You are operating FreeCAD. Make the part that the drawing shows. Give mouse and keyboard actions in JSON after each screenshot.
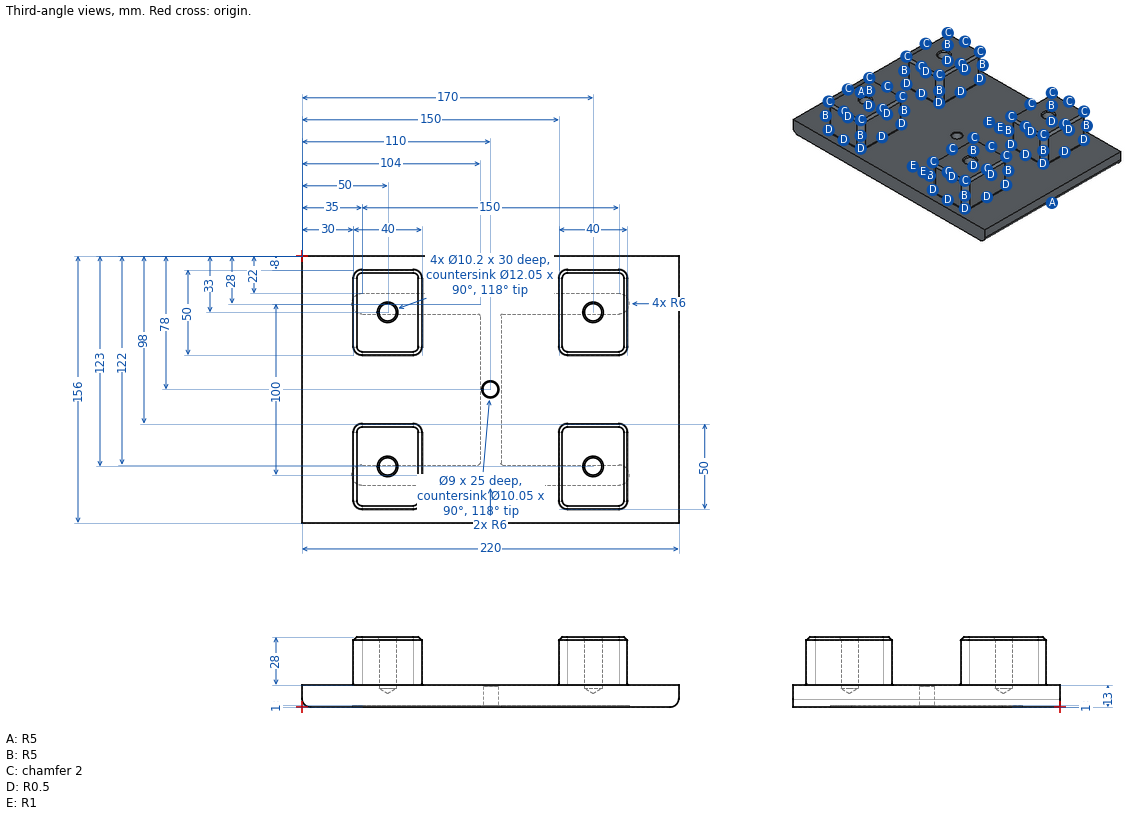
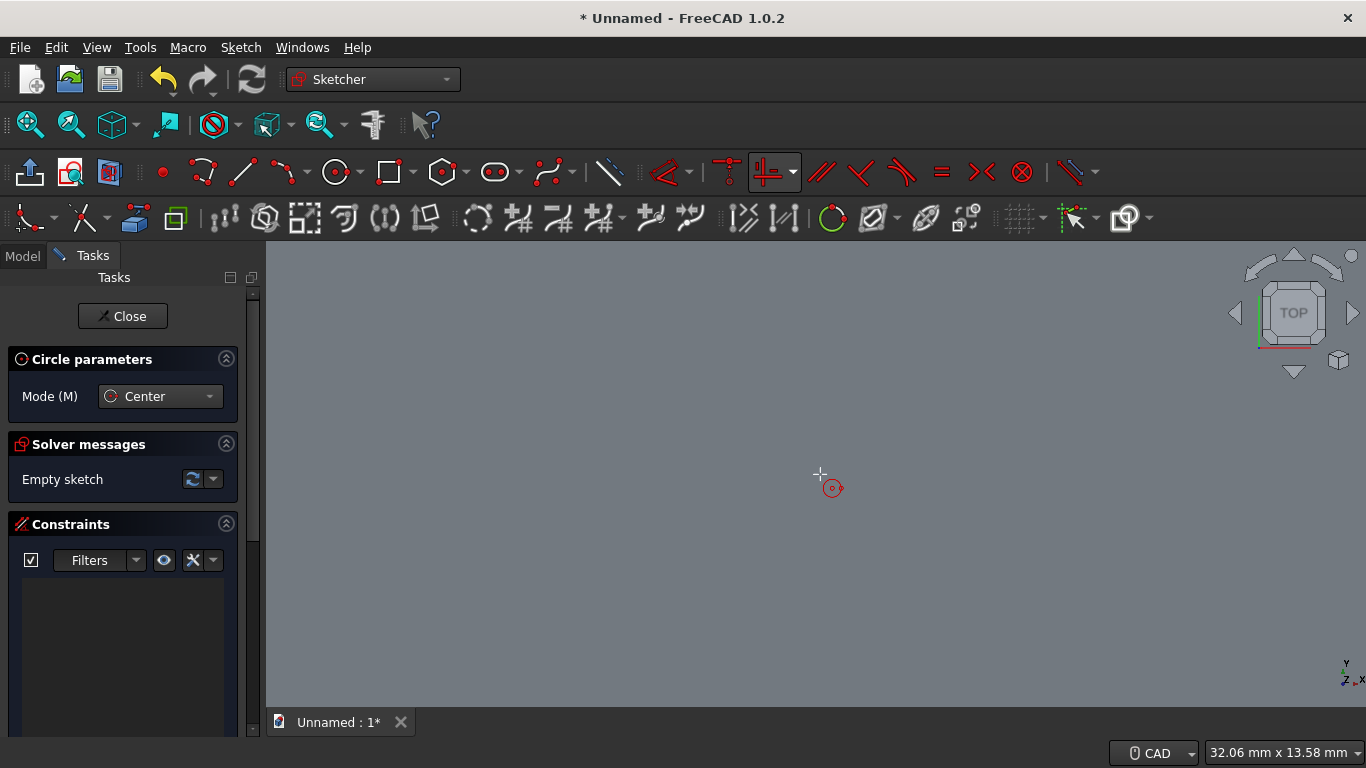
{"action": "left_click", "coordinate": [730, 464]}
{"action": "left_click", "coordinate": [839, 355]}
{"action": "key", "text": "Escape"}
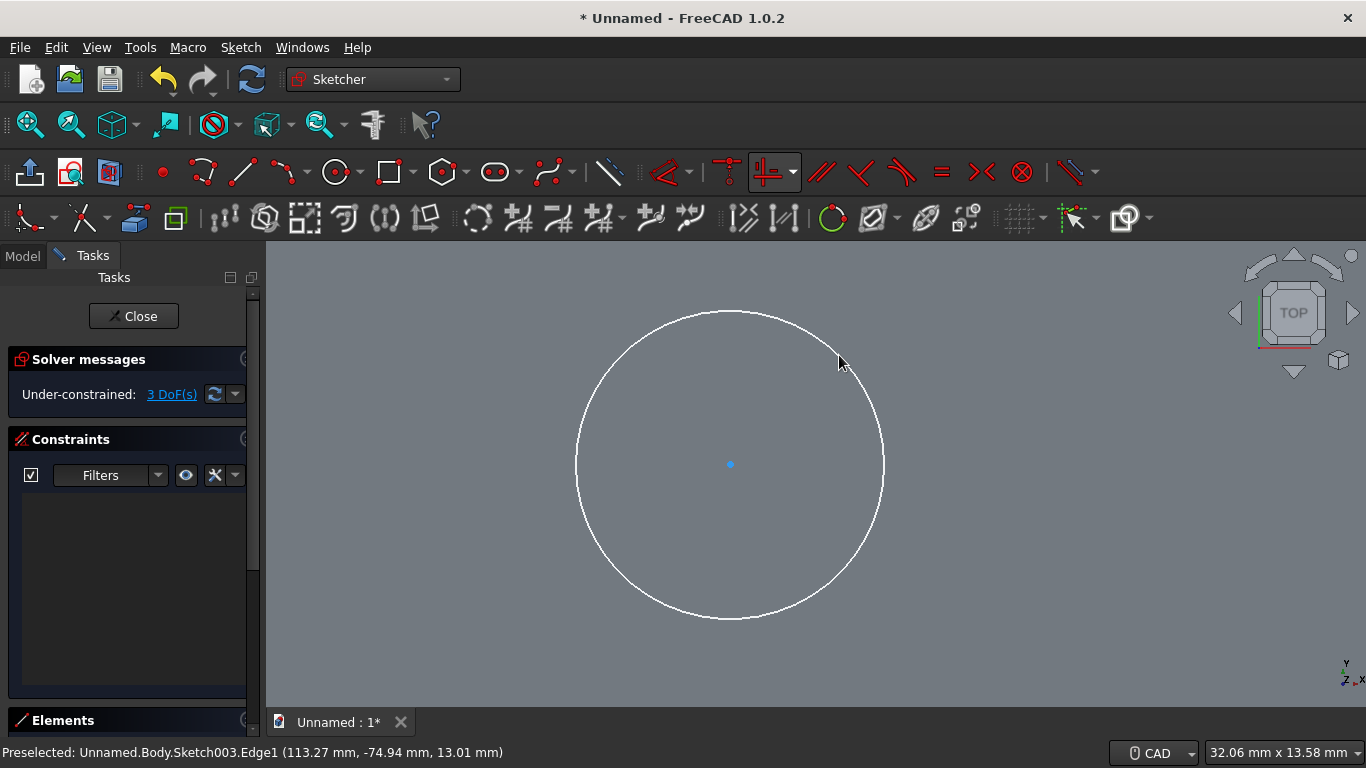
{"action": "left_click", "coordinate": [664, 172]}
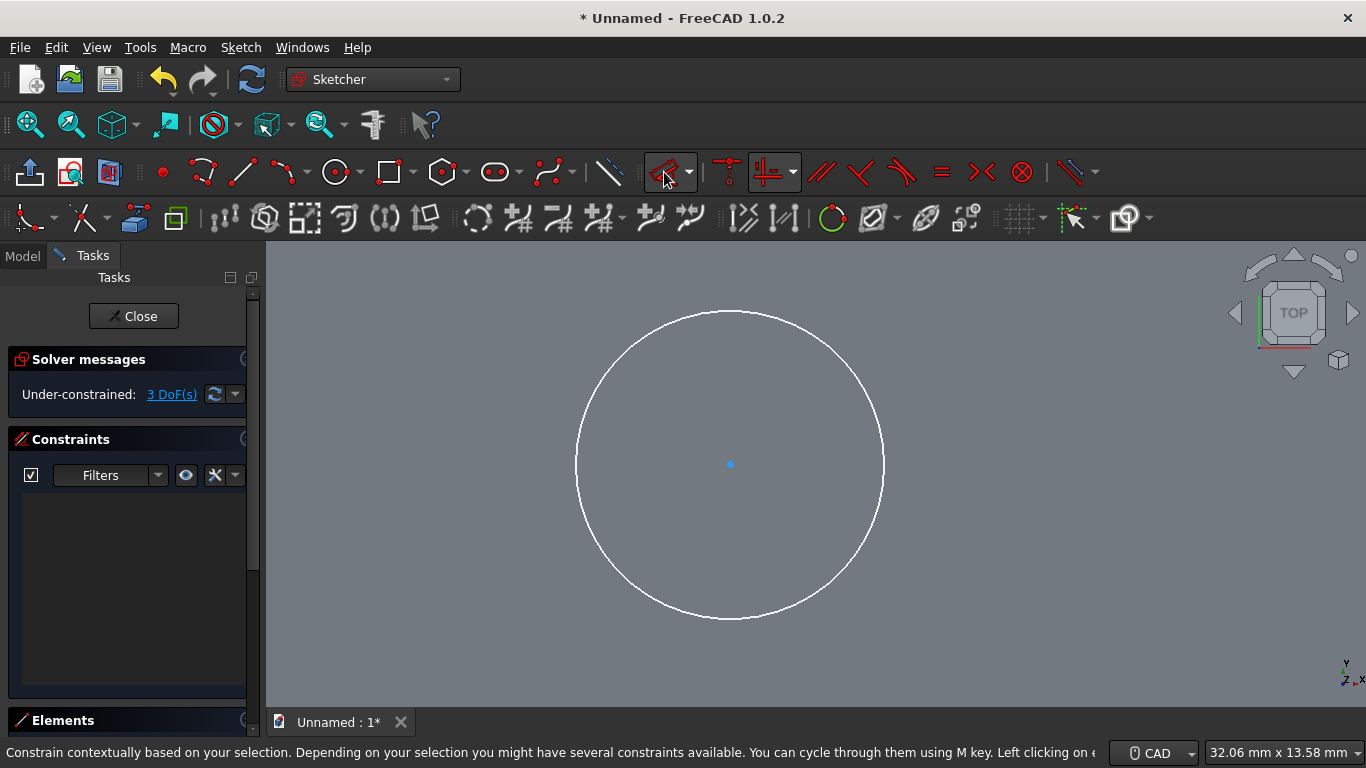
{"action": "left_click", "coordinate": [839, 356]}
{"action": "left_click", "coordinate": [862, 333]}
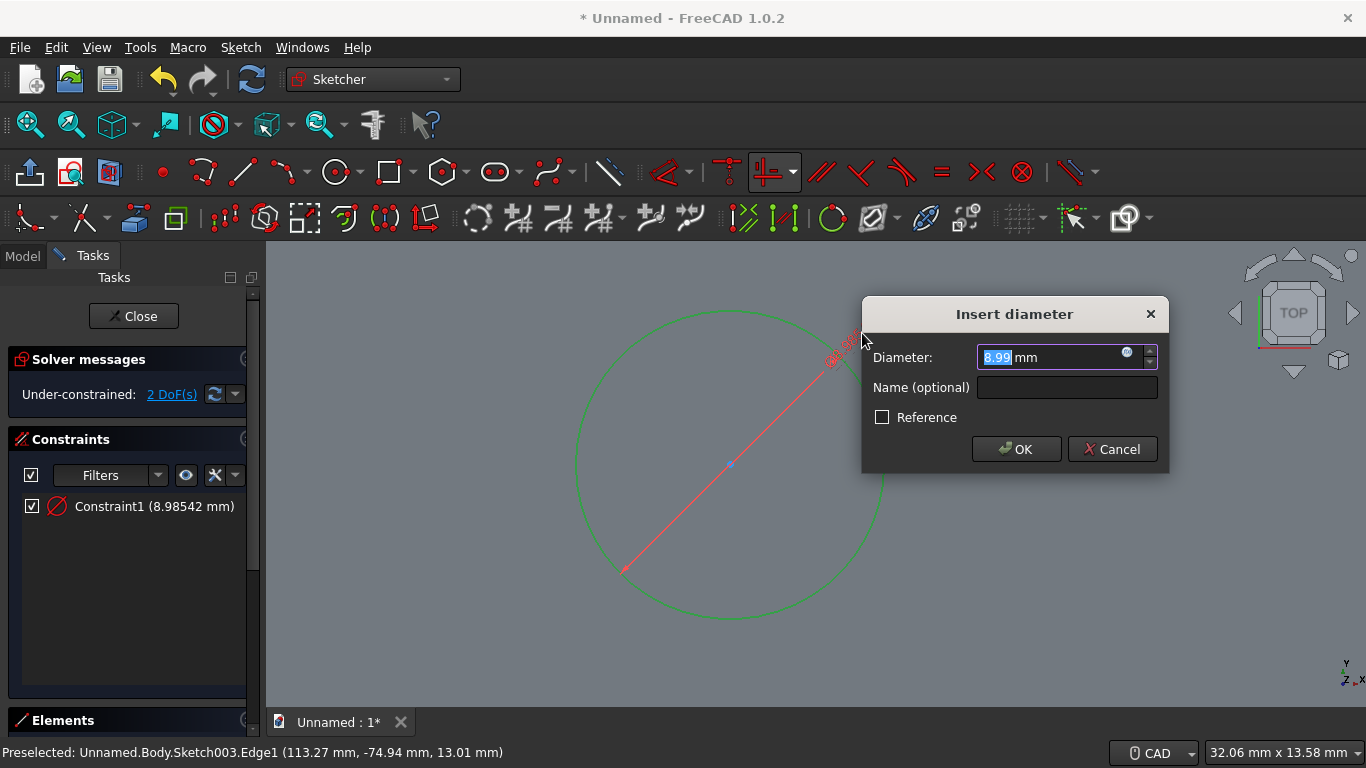
{"action": "type", "text": "9"}
{"action": "key", "text": "Return"}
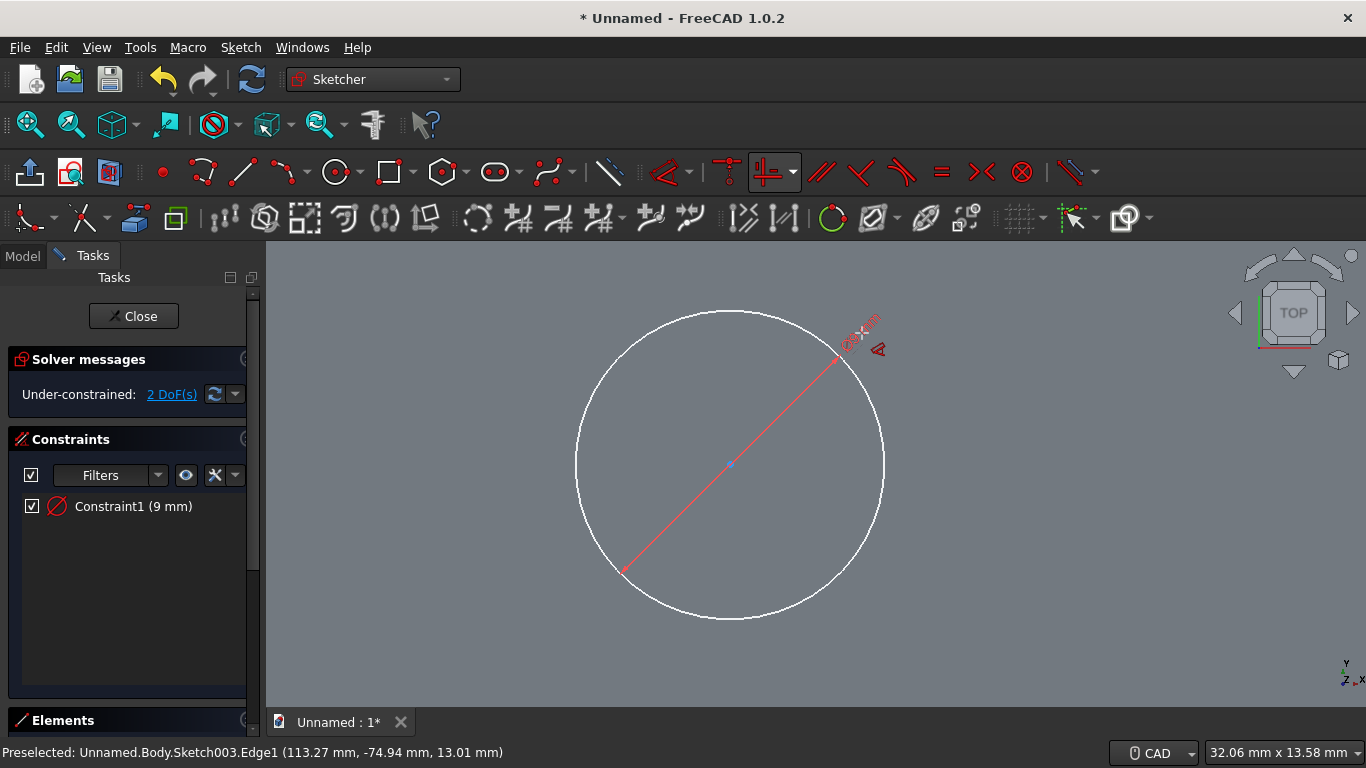
{"action": "left_click", "coordinate": [730, 465]}
{"action": "left_click", "coordinate": [764, 367]}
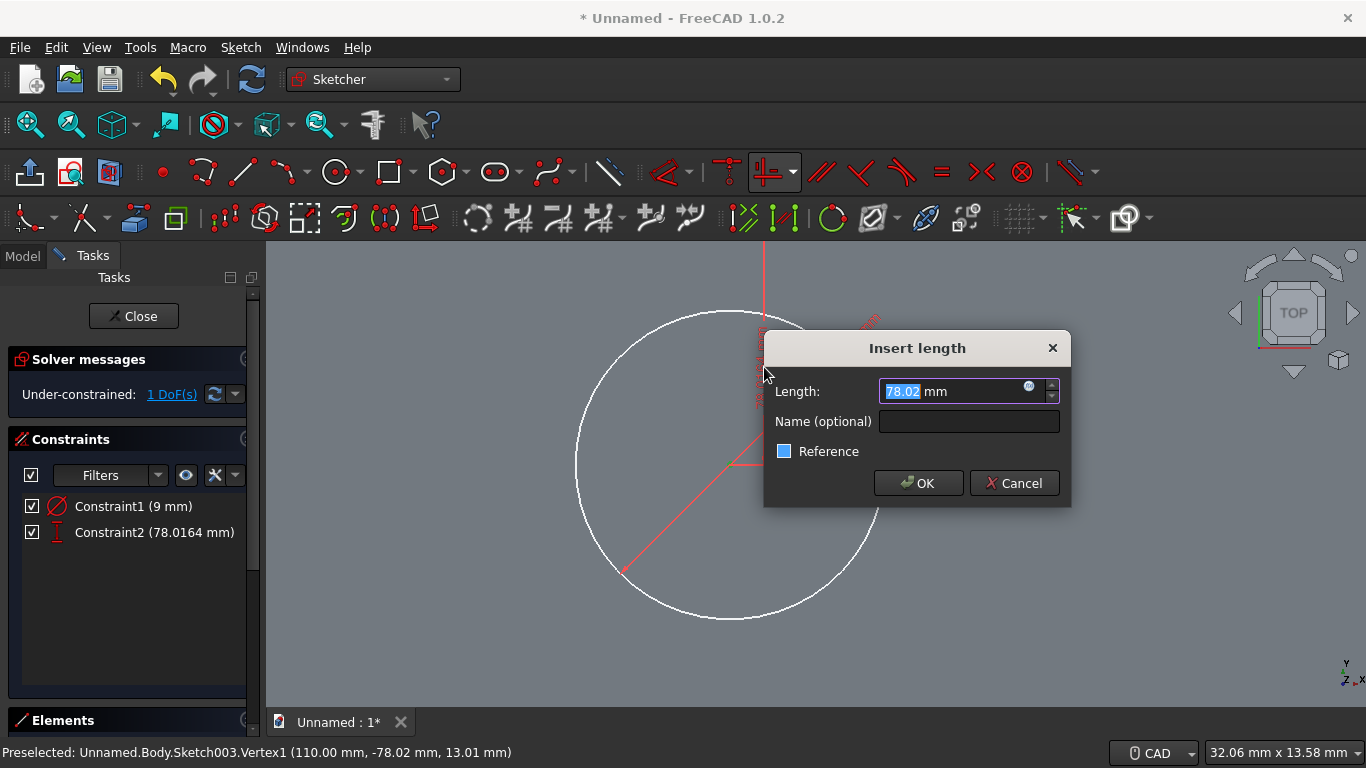
{"action": "type", "text": "78"}
{"action": "key", "text": "Return"}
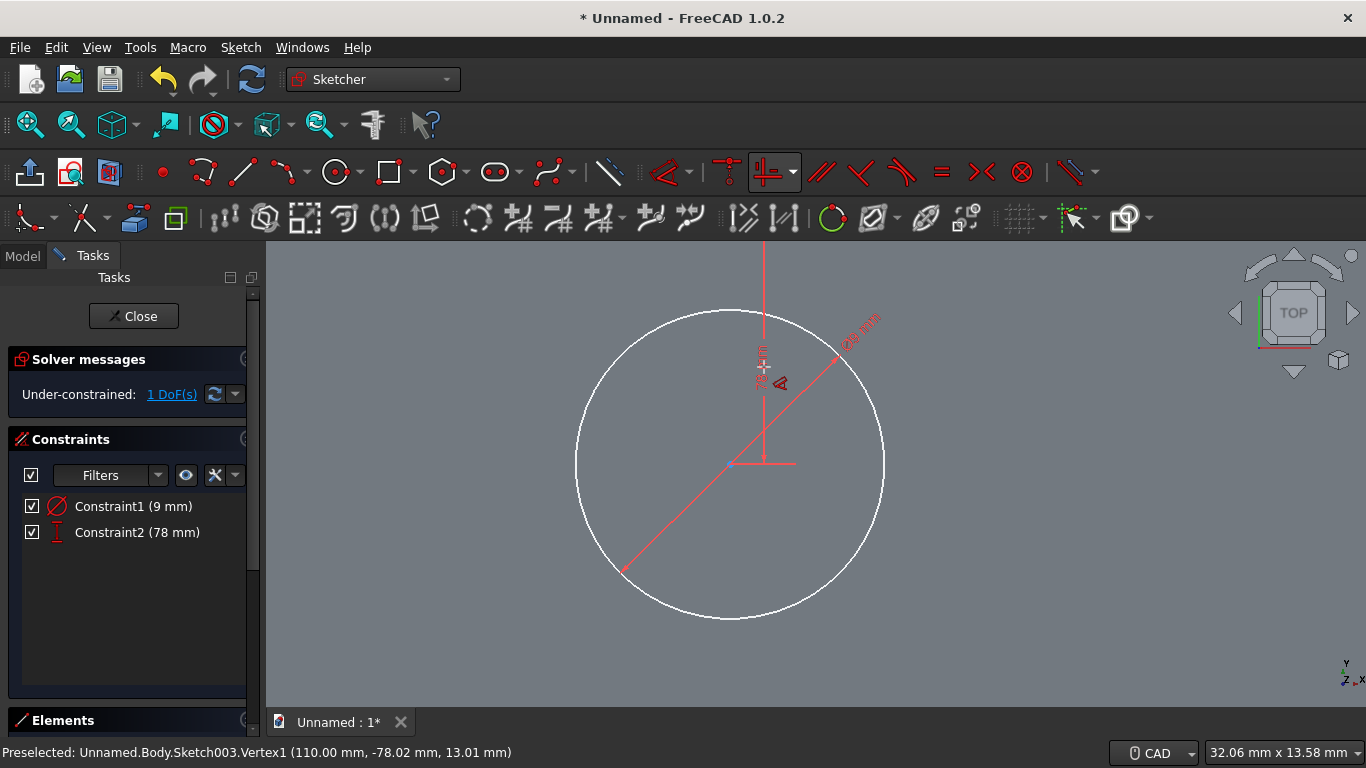
{"action": "left_click", "coordinate": [730, 464]}
{"action": "left_click", "coordinate": [512, 498]}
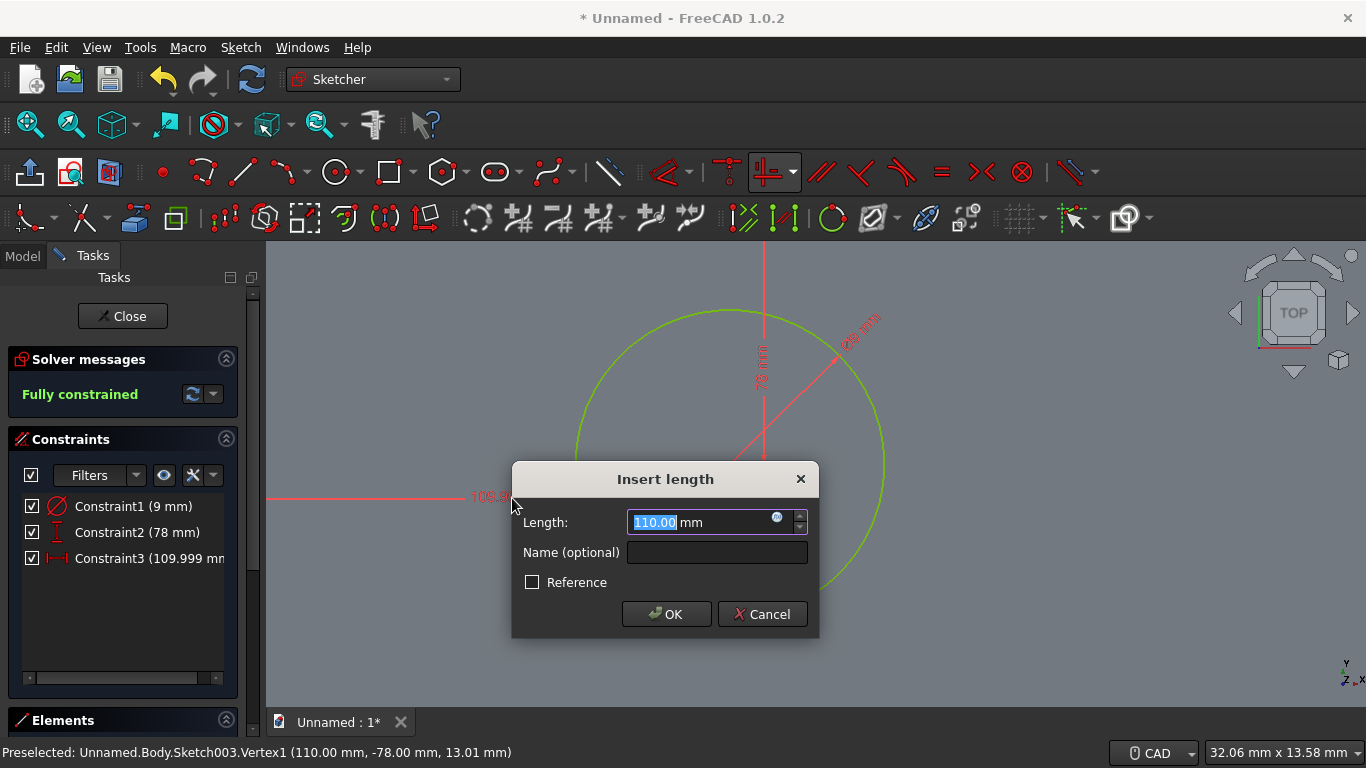
{"action": "type", "text": "110"}
{"action": "key", "text": "Return"}
{"action": "key", "text": "Escape"}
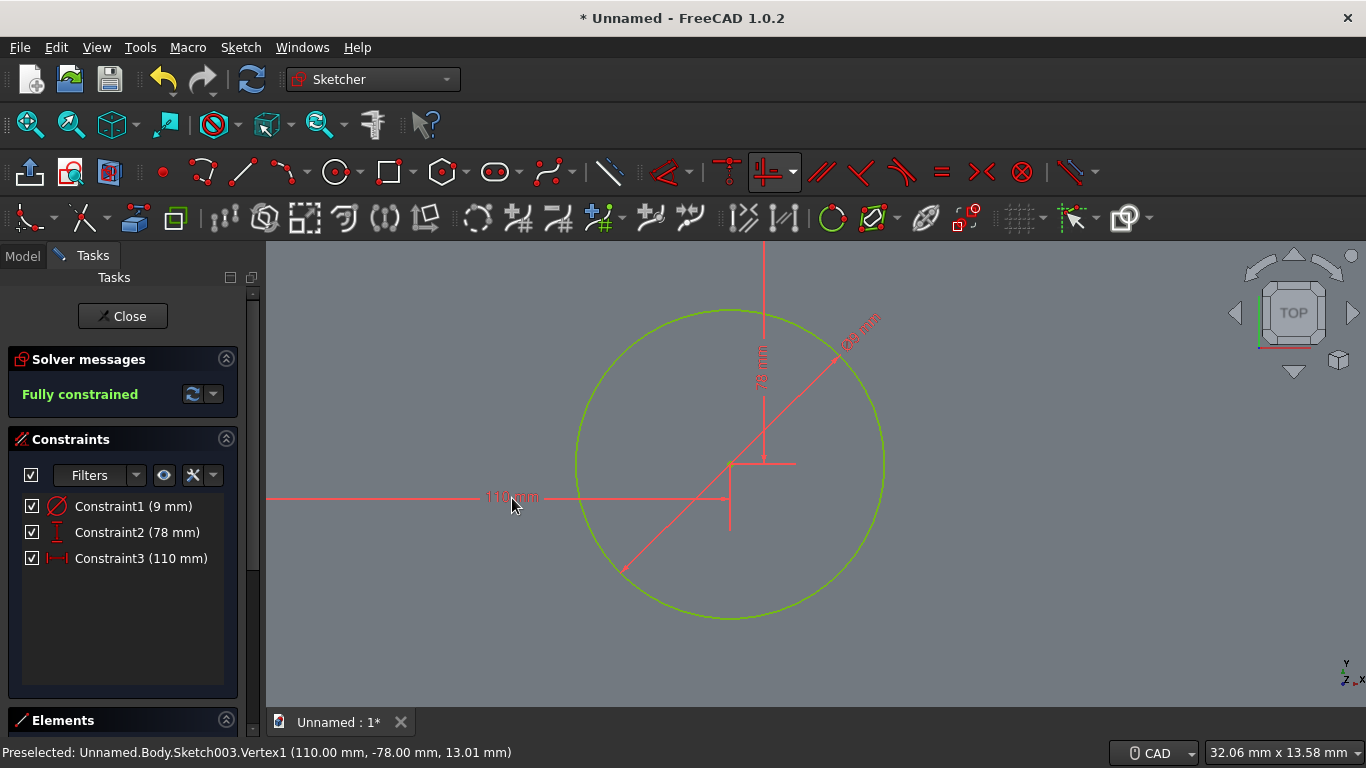
{"action": "left_click", "coordinate": [123, 316]}